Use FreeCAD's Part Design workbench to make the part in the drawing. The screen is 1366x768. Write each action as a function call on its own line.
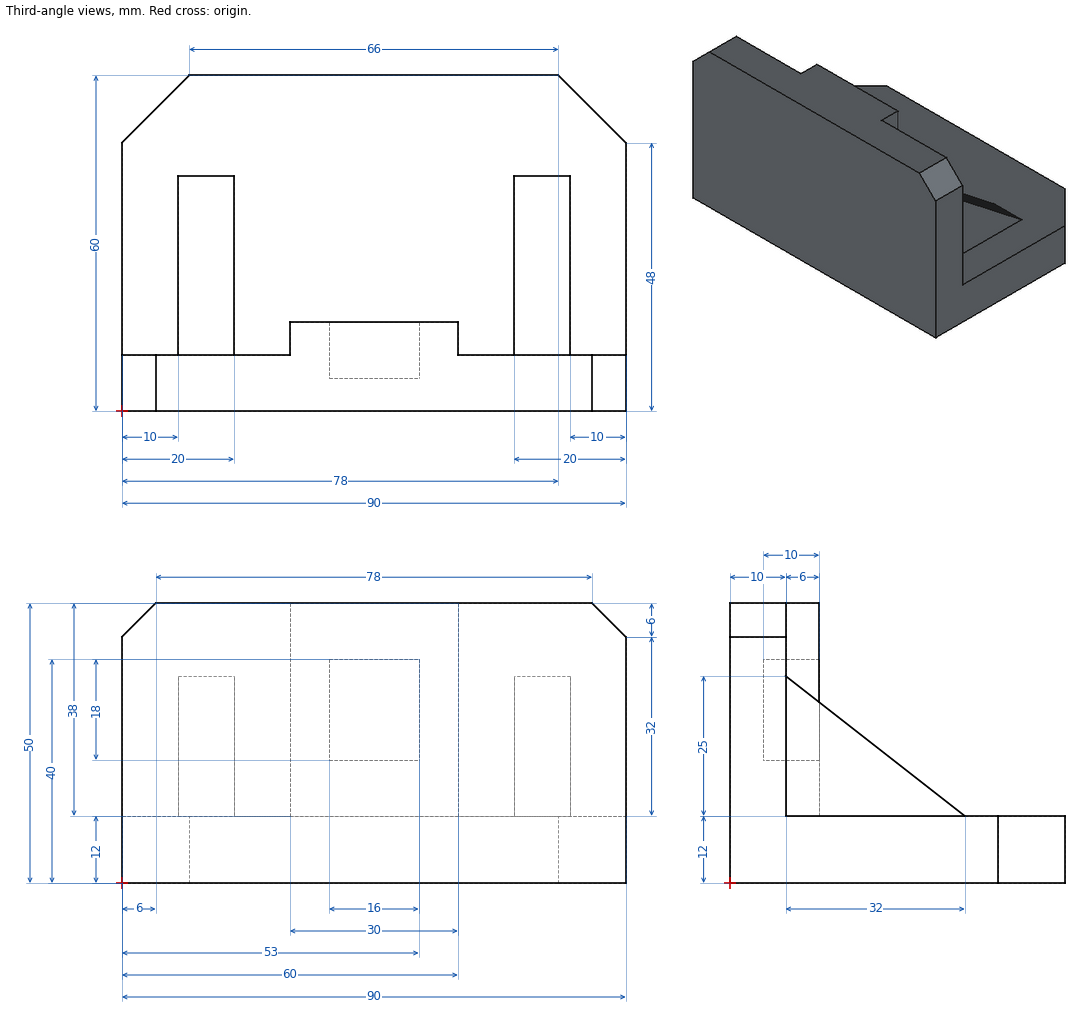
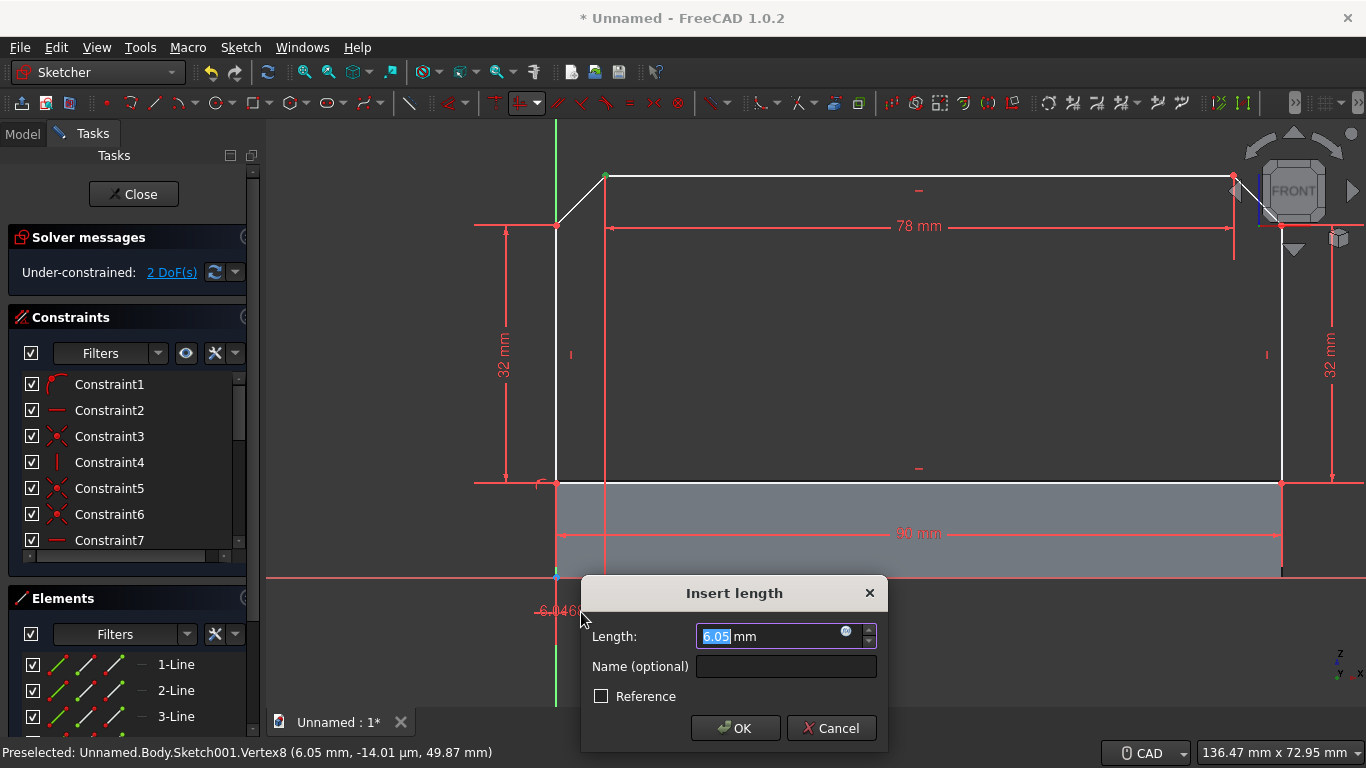
text(6)
key(Return)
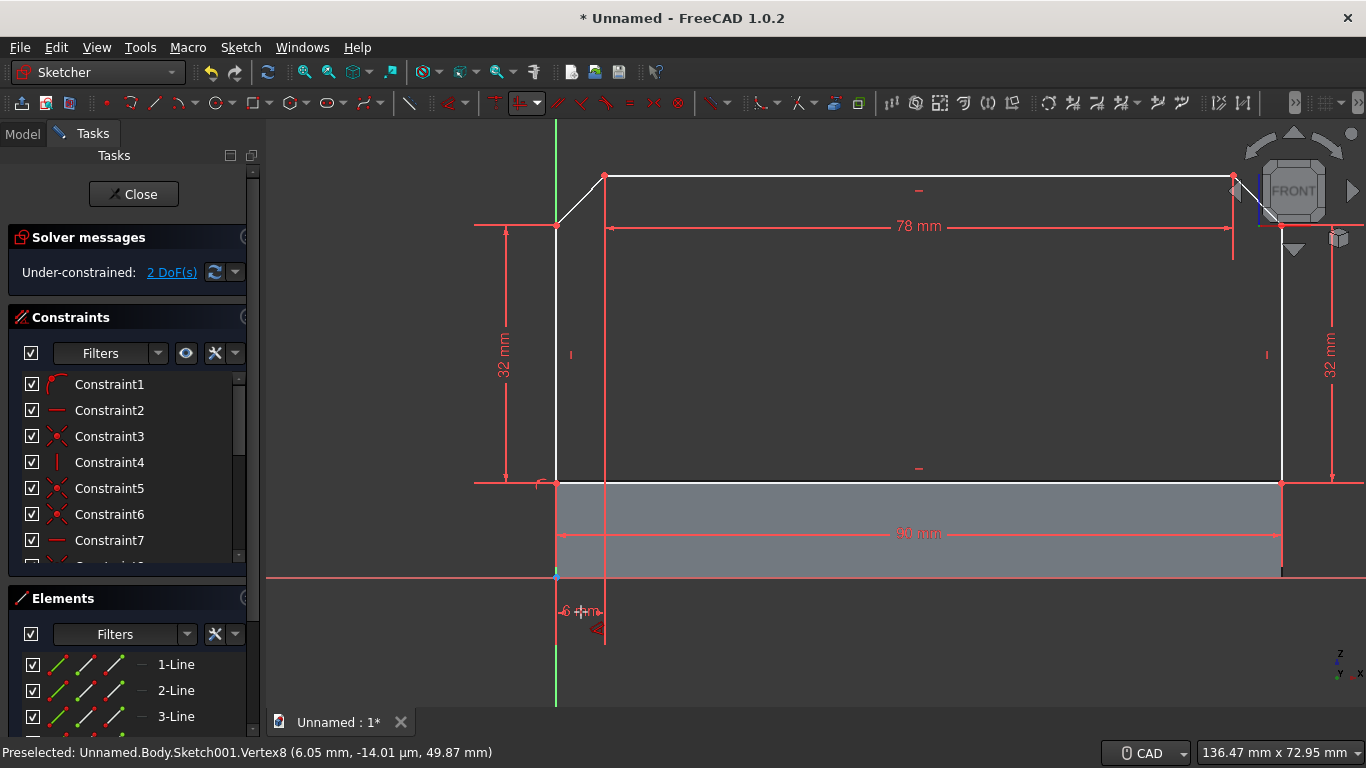
scroll(294, 578, down, 1)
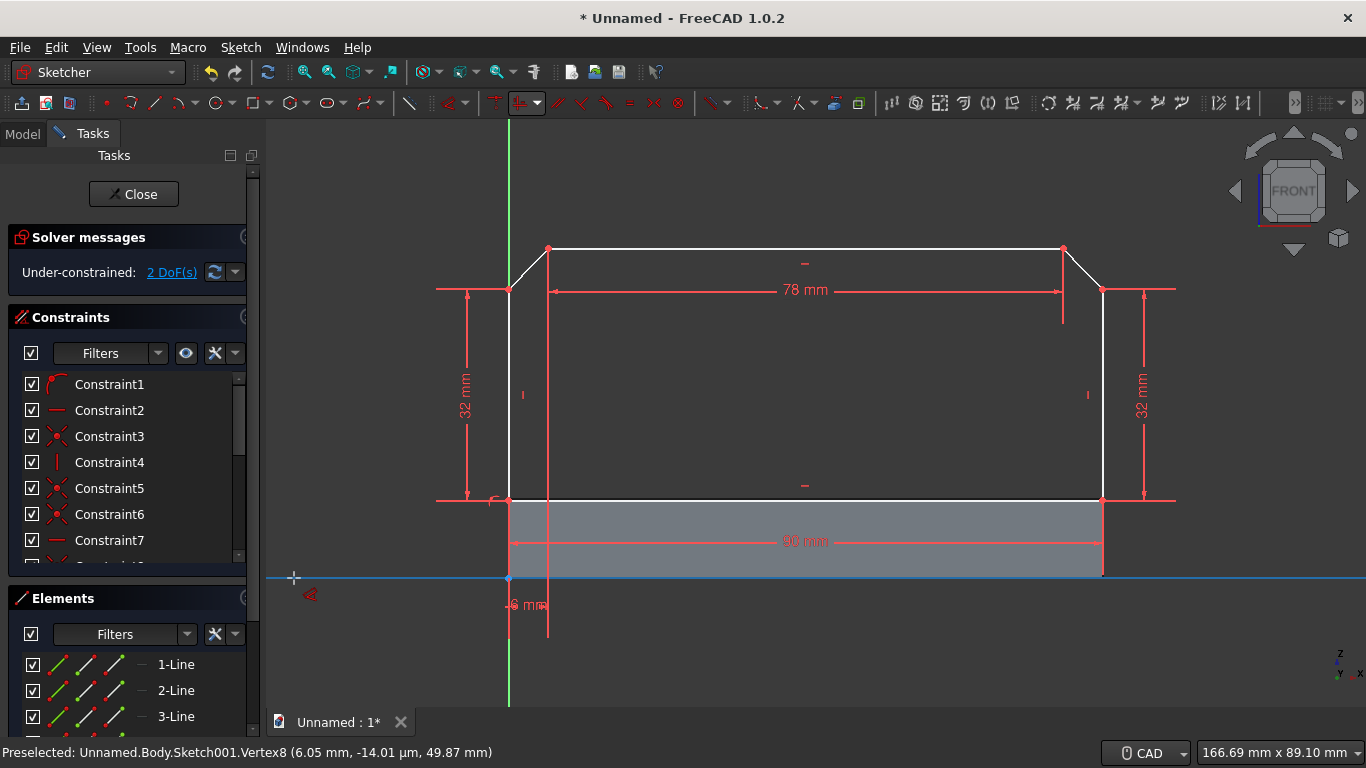
click(1091, 277)
click(1137, 269)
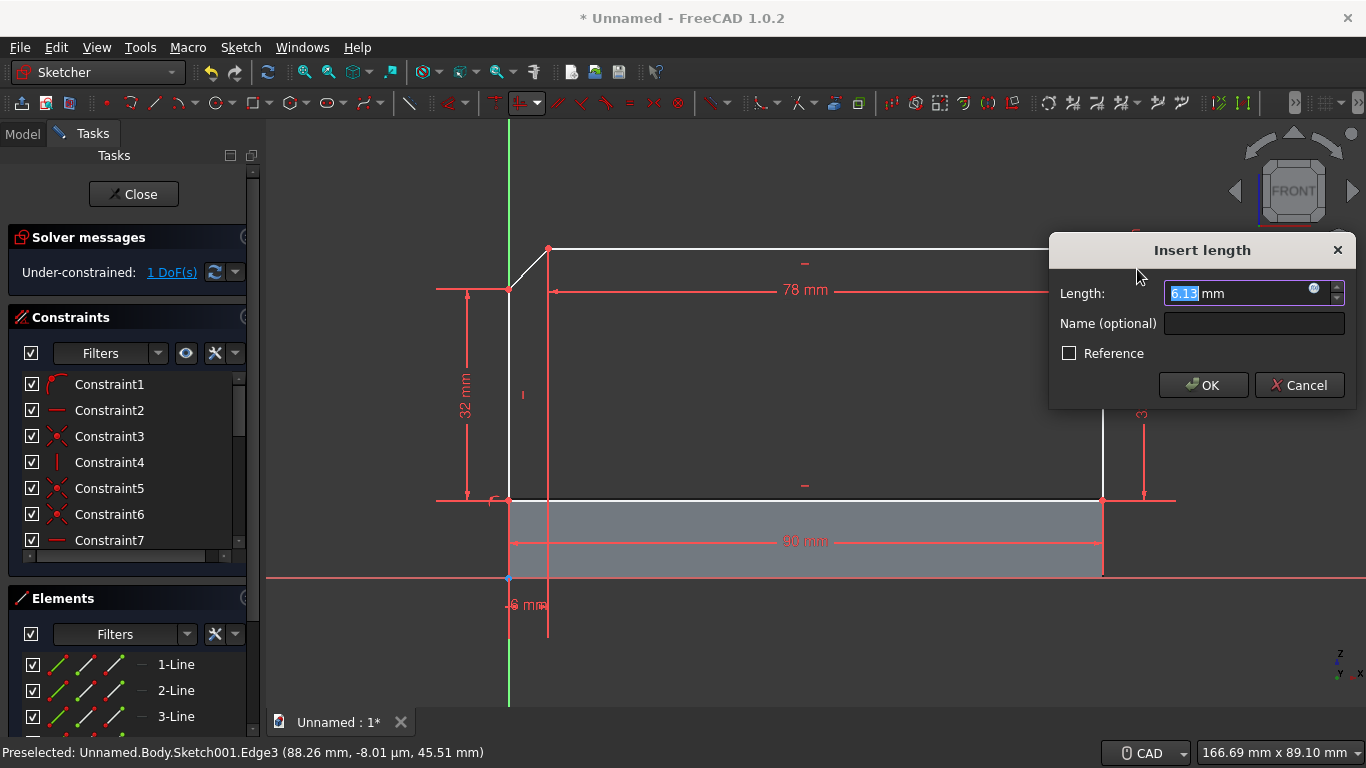
text(6)
key(Return)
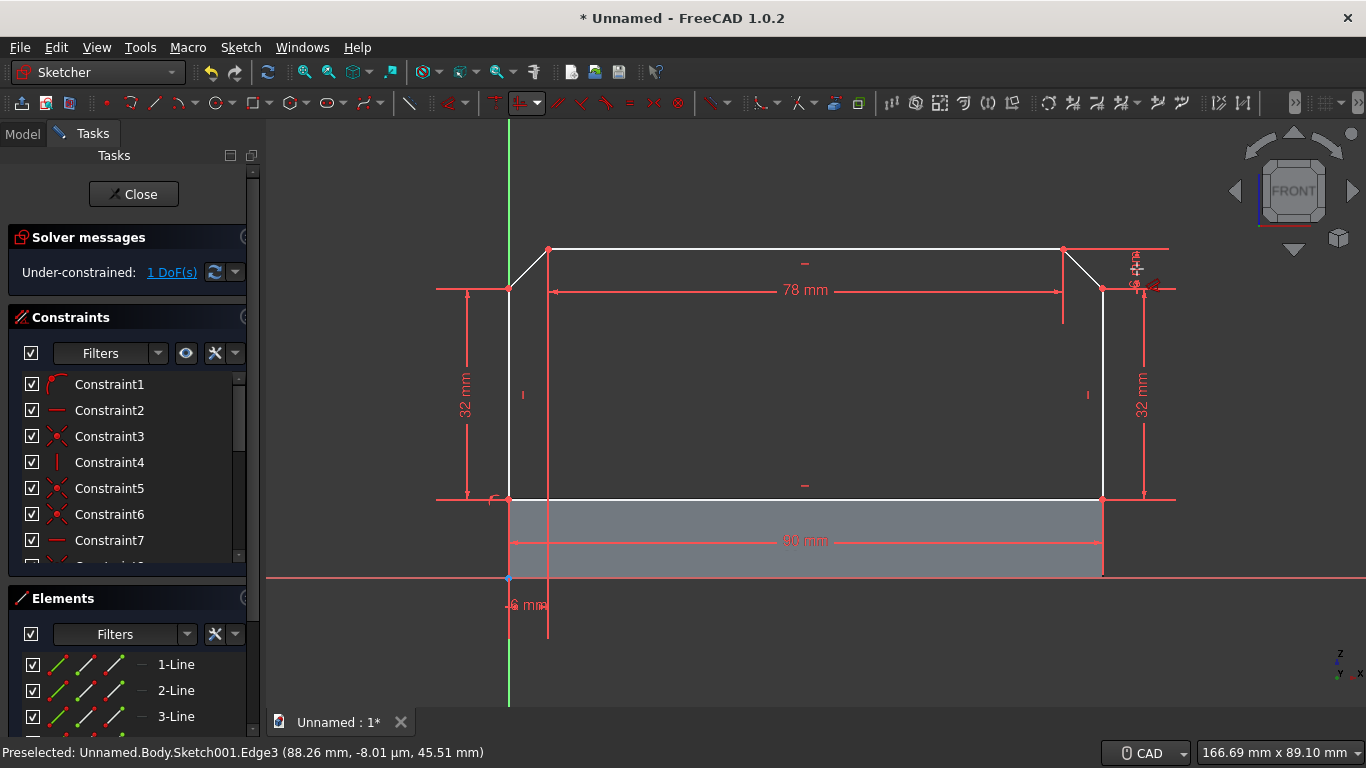
click(509, 500)
click(475, 539)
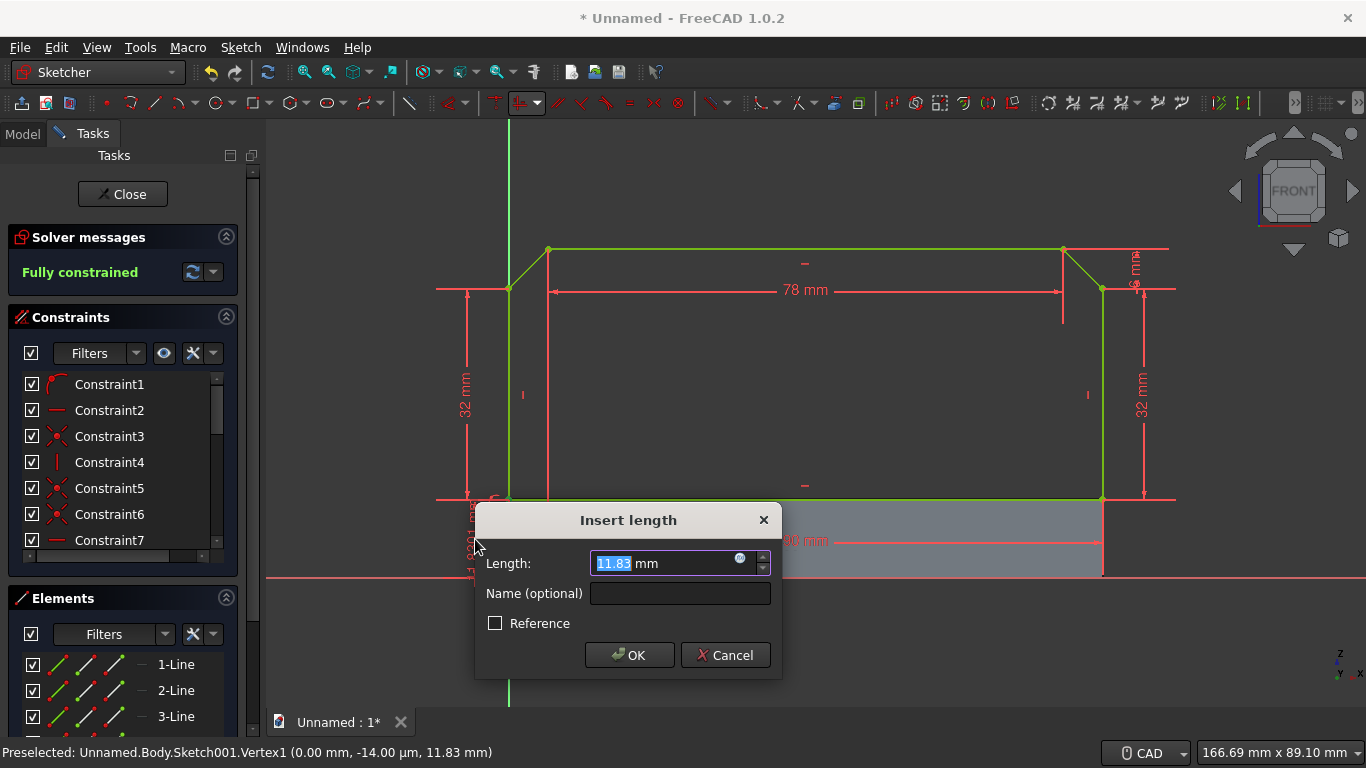
text(12)
key(Return)
key(Escape)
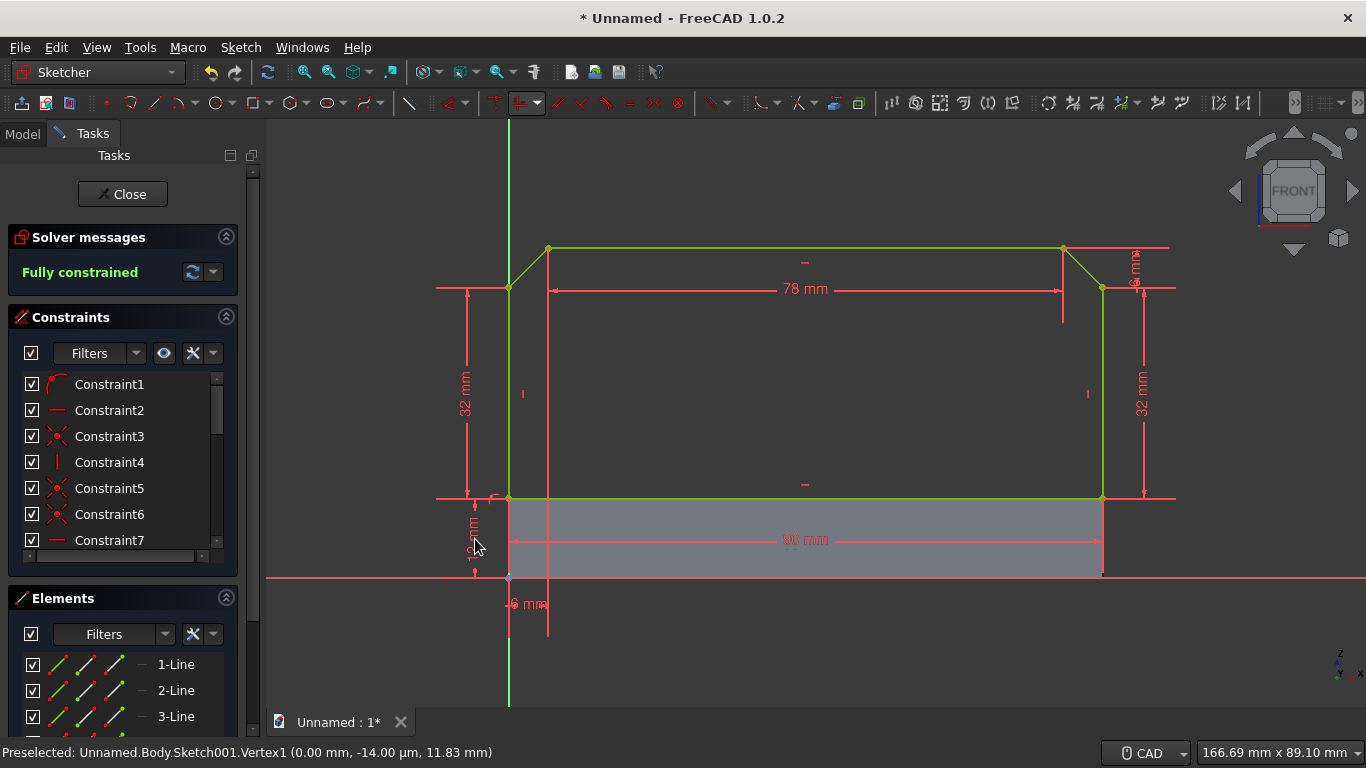
click(123, 194)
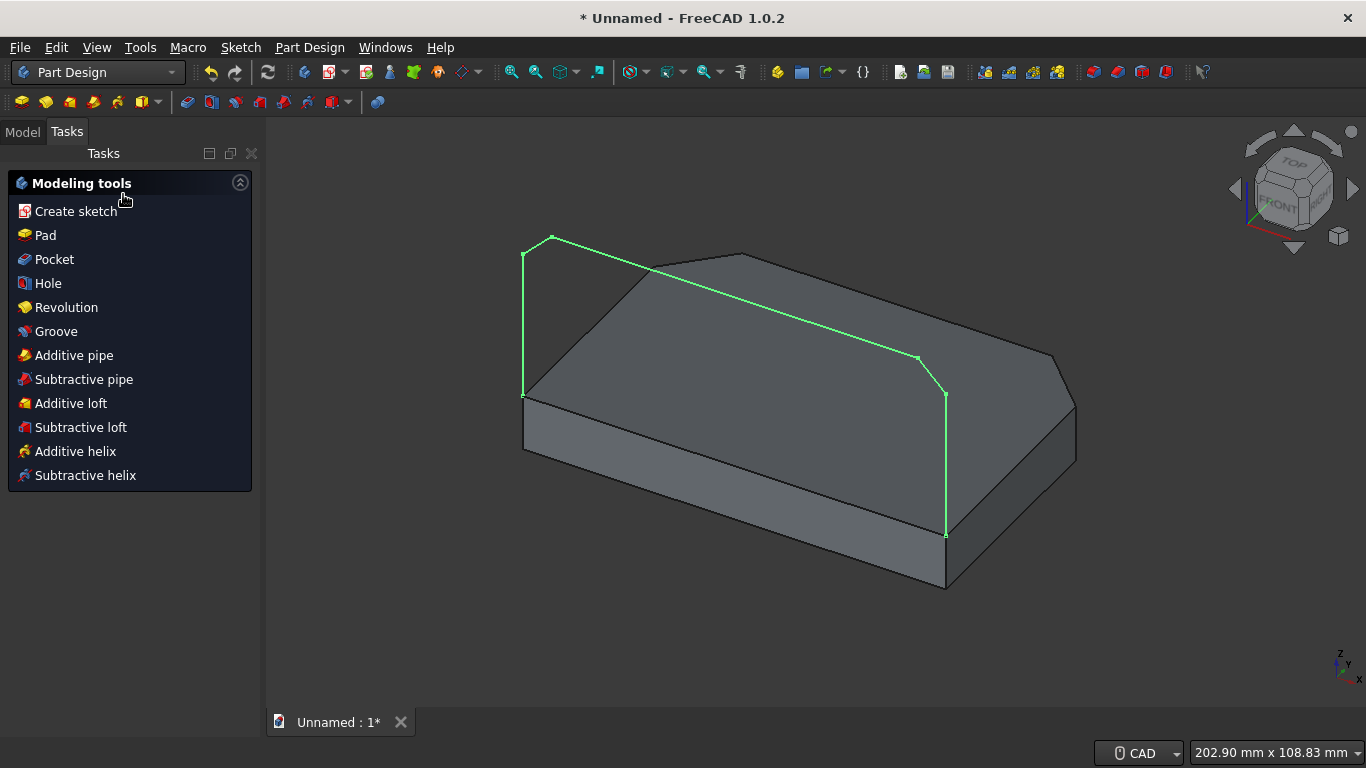
click(22, 102)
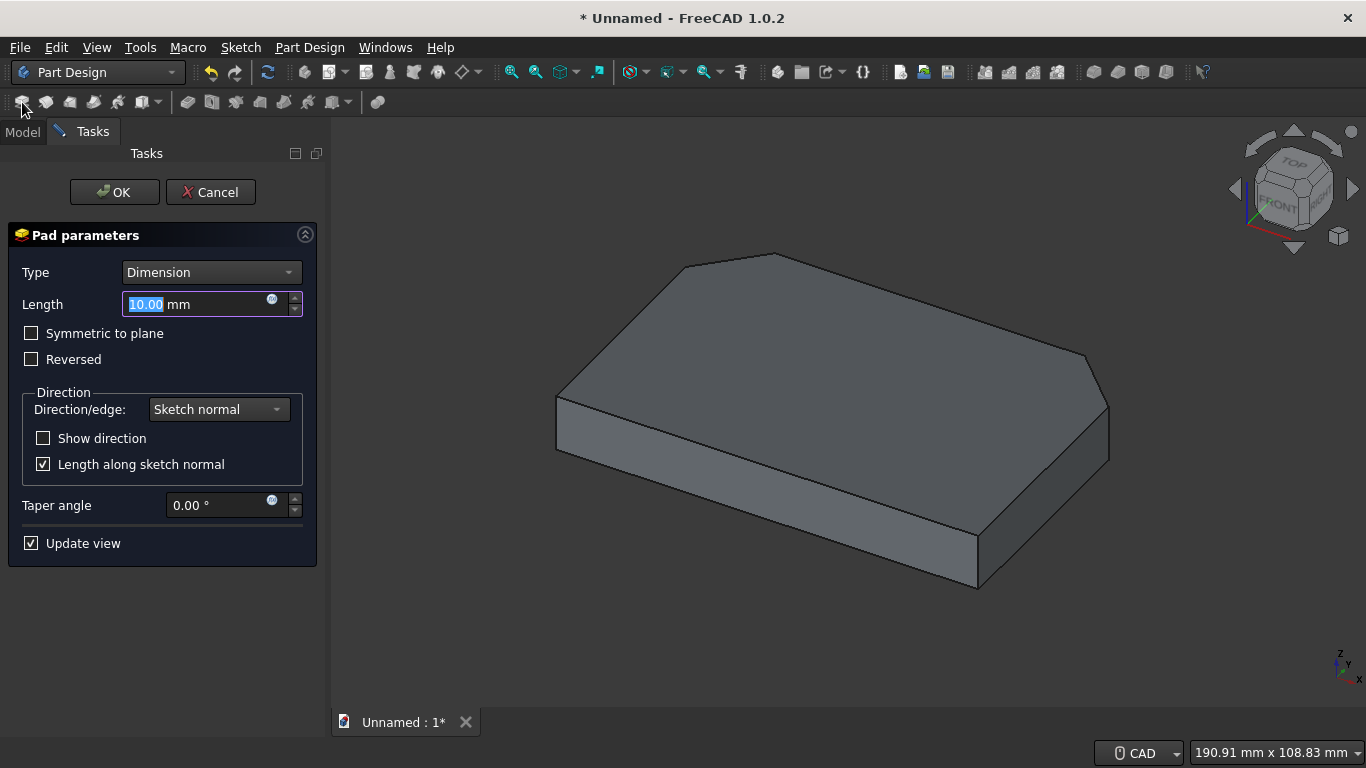
text(10)
key(Tab)